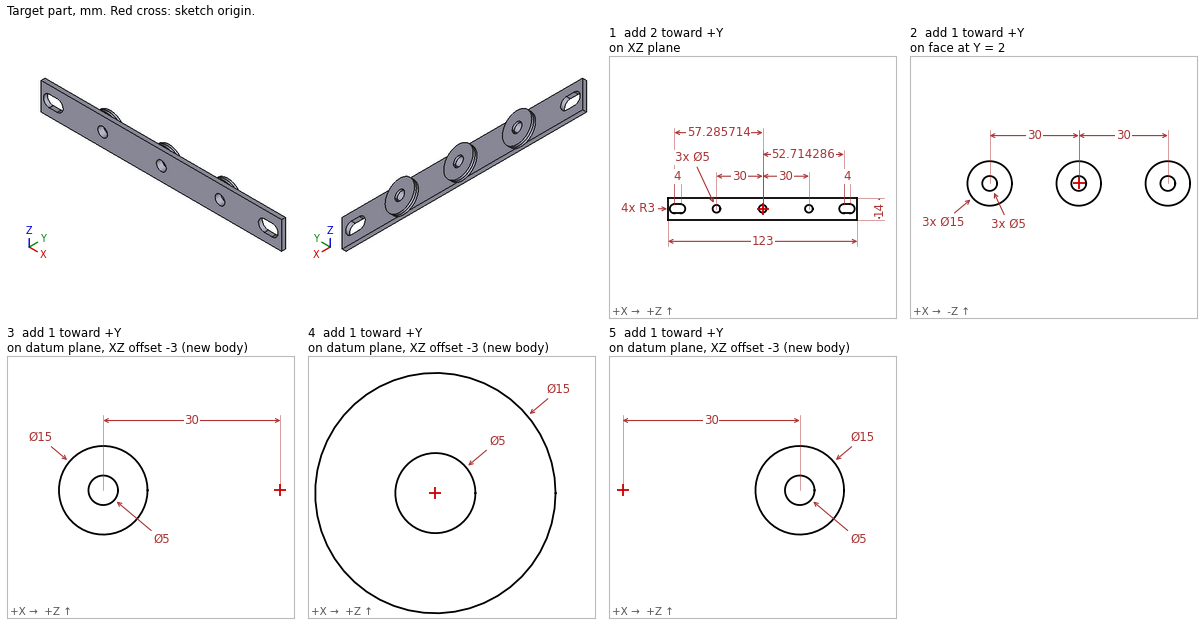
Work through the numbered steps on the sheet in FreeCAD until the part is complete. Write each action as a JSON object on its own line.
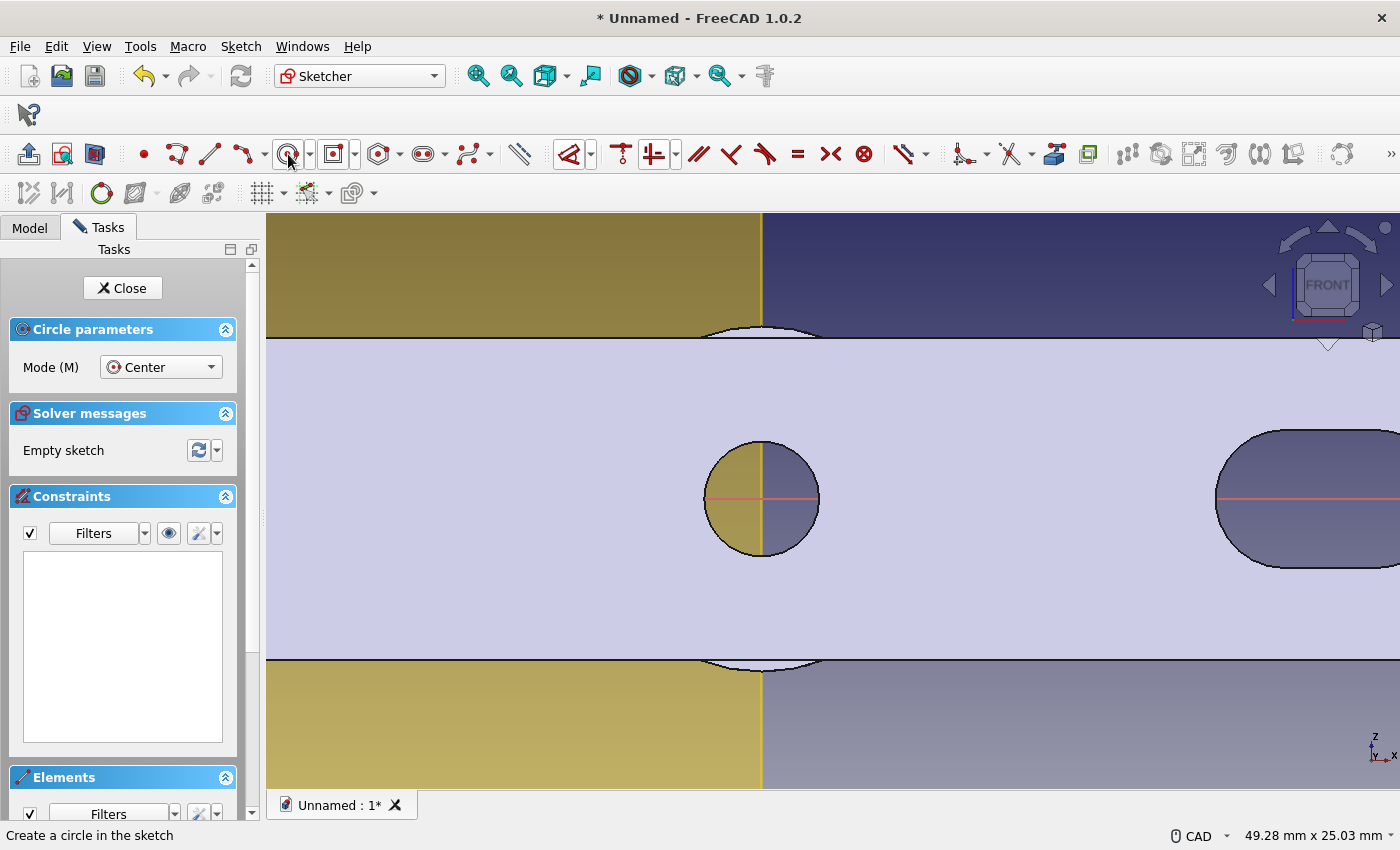
{"action": "left_click", "coordinate": [762, 499]}
{"action": "left_click", "coordinate": [884, 377]}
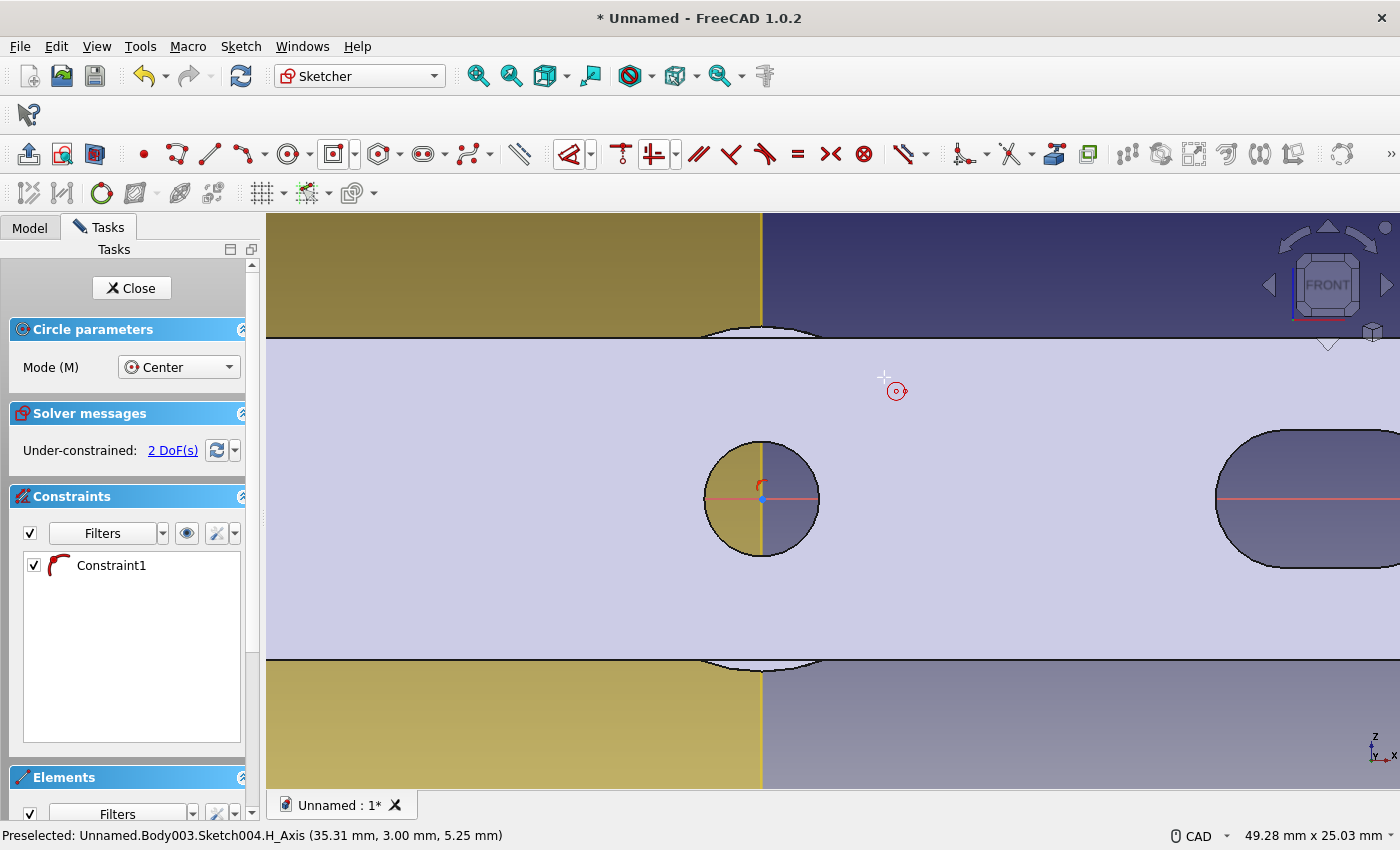
{"action": "left_click", "coordinate": [762, 499]}
{"action": "left_click", "coordinate": [802, 458]}
{"action": "key", "text": "Escape"}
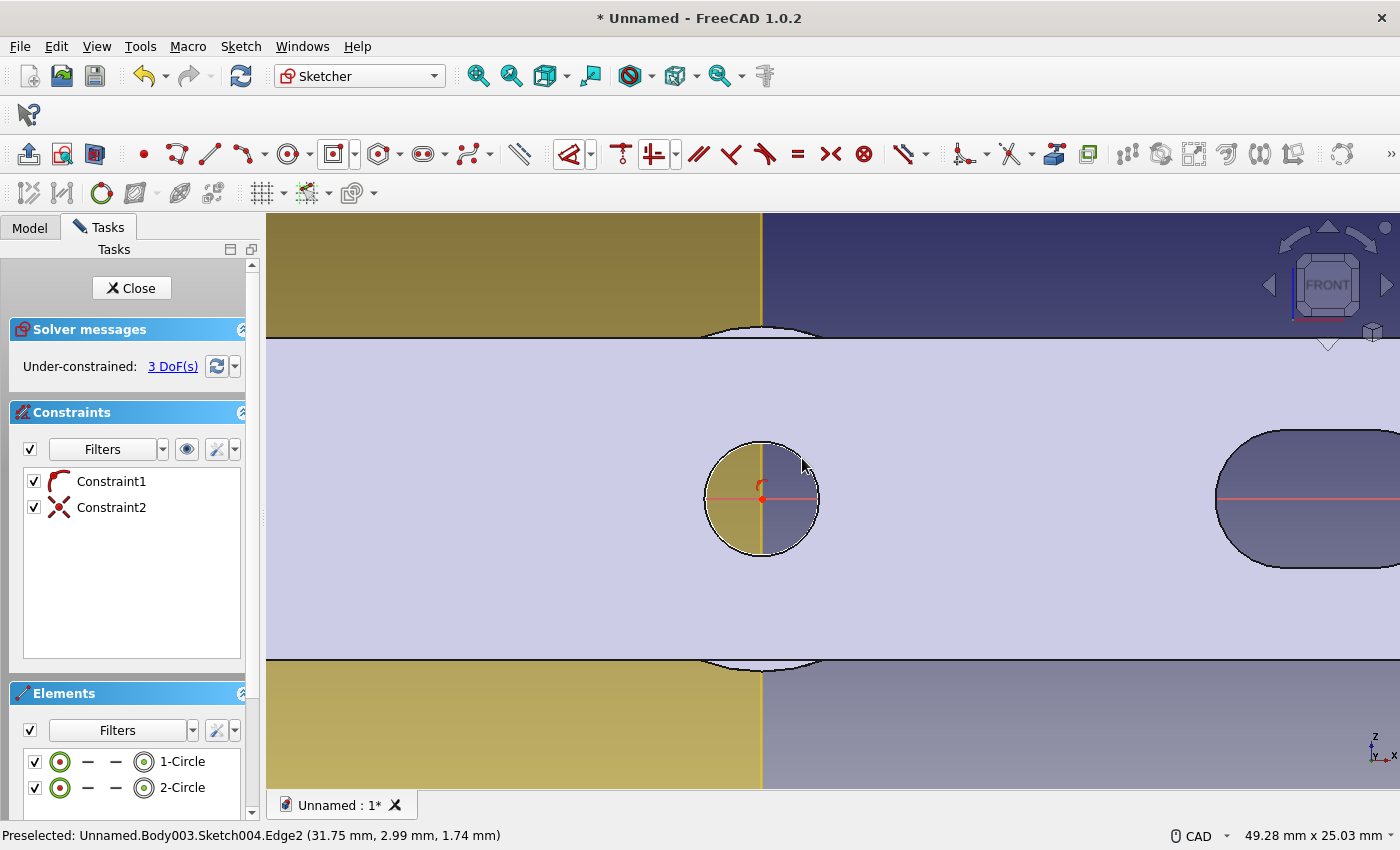
{"action": "left_click", "coordinate": [883, 377]}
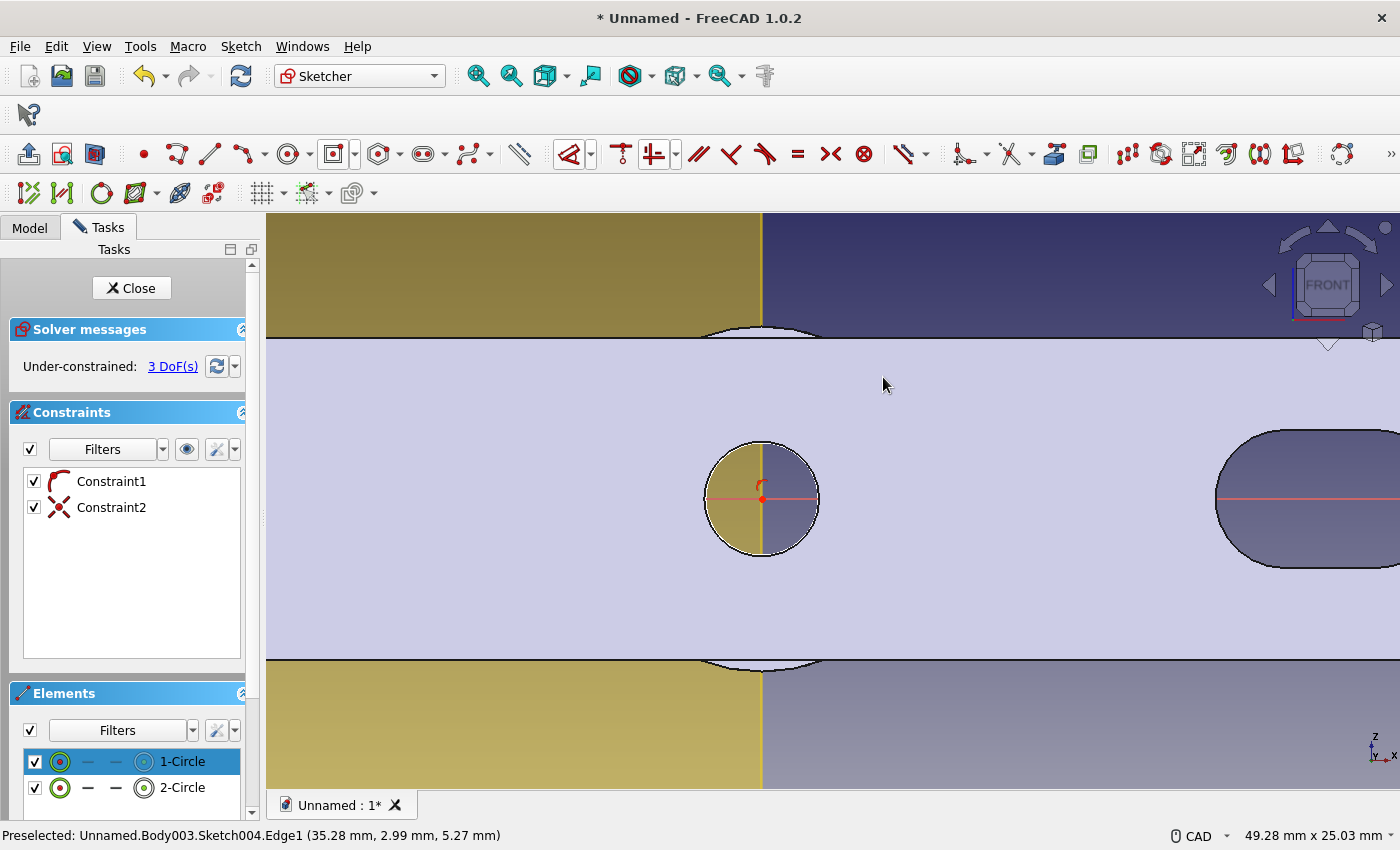
{"action": "left_click", "coordinate": [590, 154]}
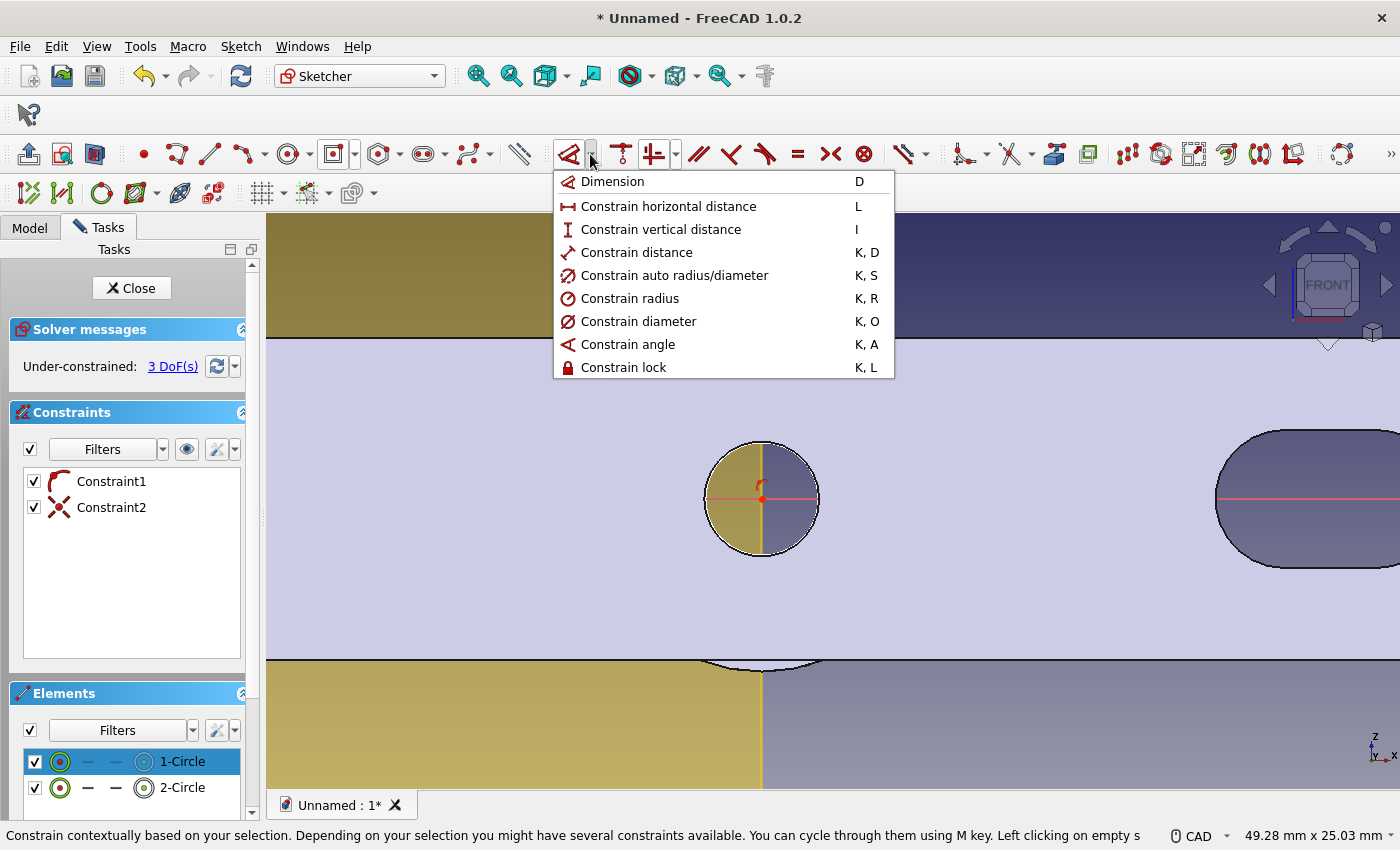
{"action": "left_click", "coordinate": [724, 322]}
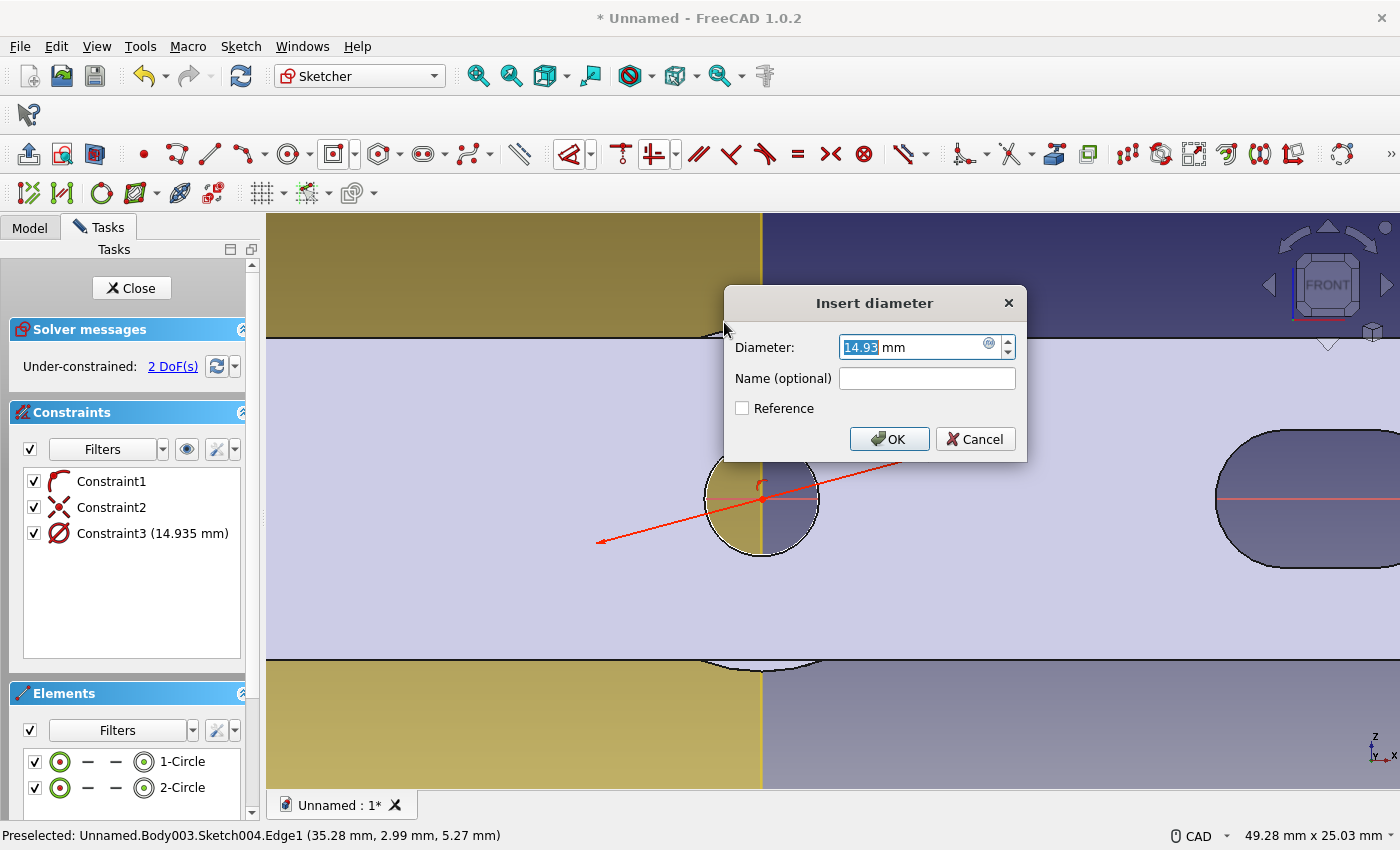
{"action": "type", "text": "15"}
{"action": "key", "text": "Return"}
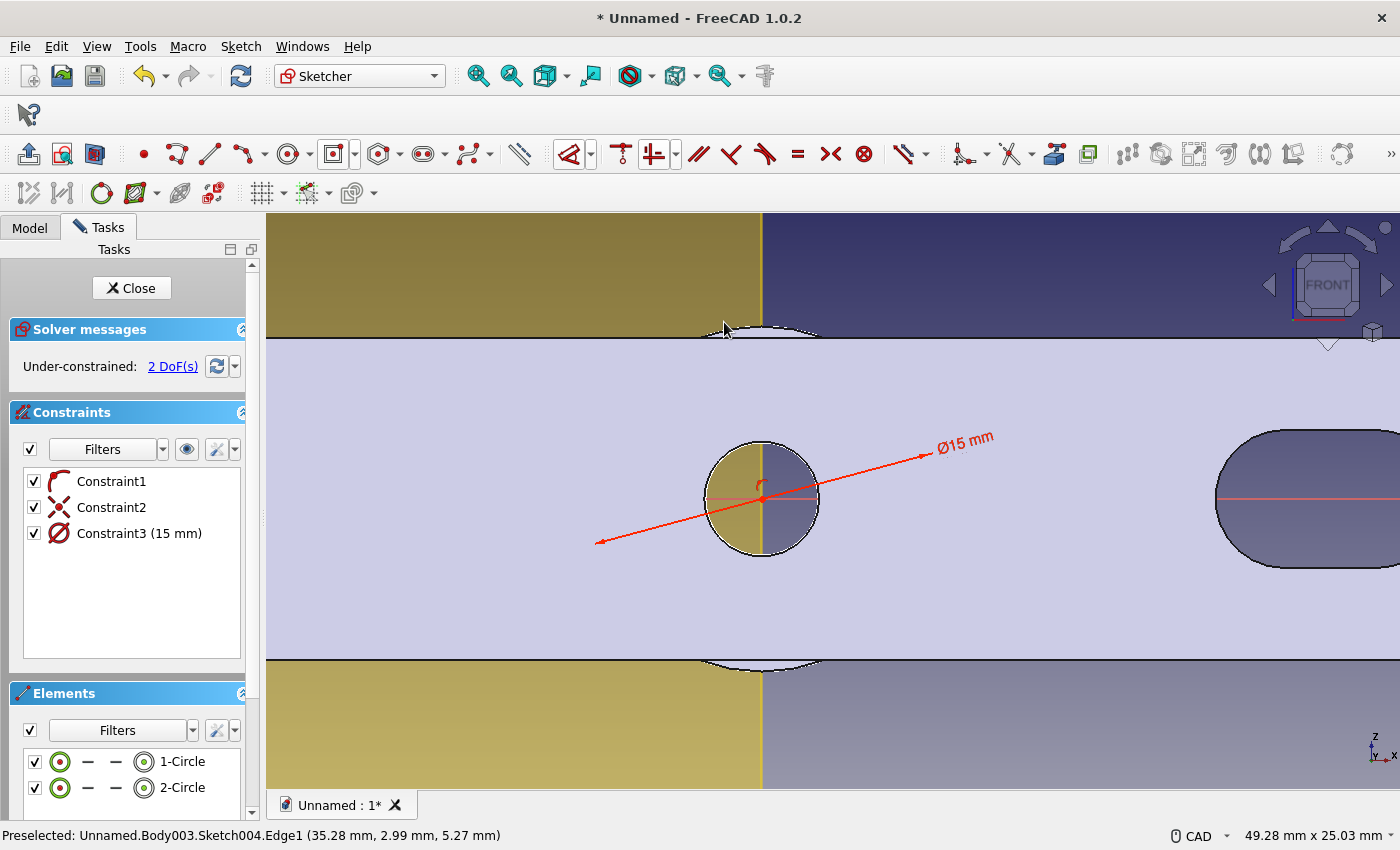
{"action": "left_click", "coordinate": [802, 459]}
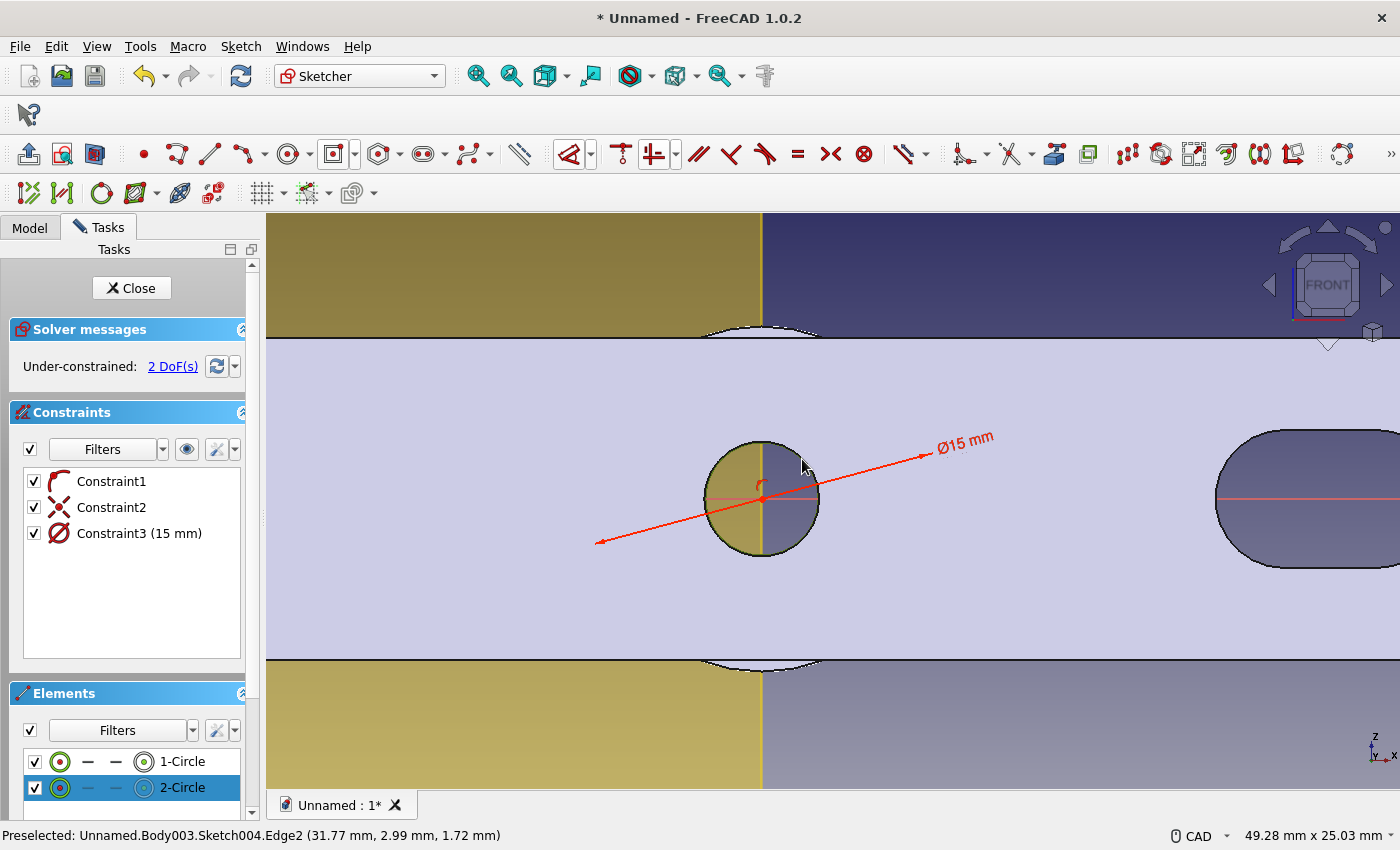
{"action": "key", "text": "k o"}